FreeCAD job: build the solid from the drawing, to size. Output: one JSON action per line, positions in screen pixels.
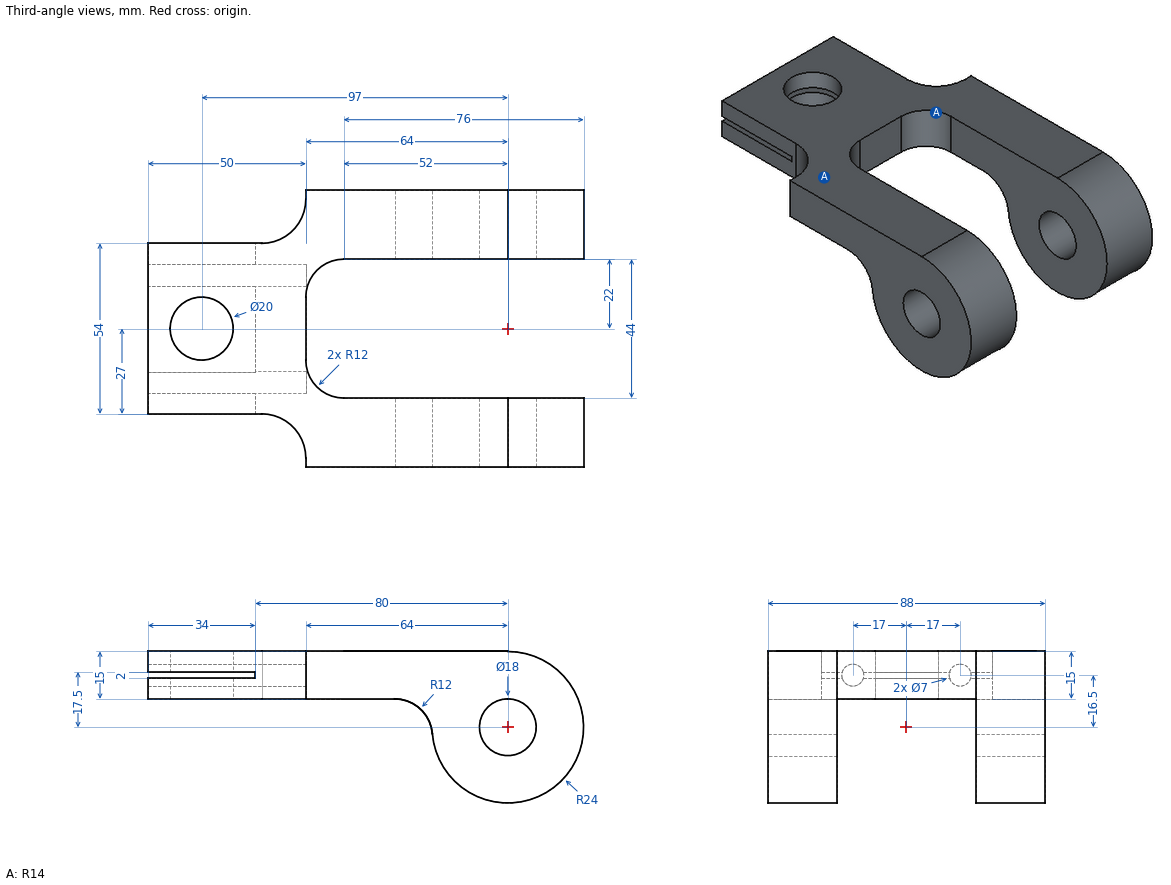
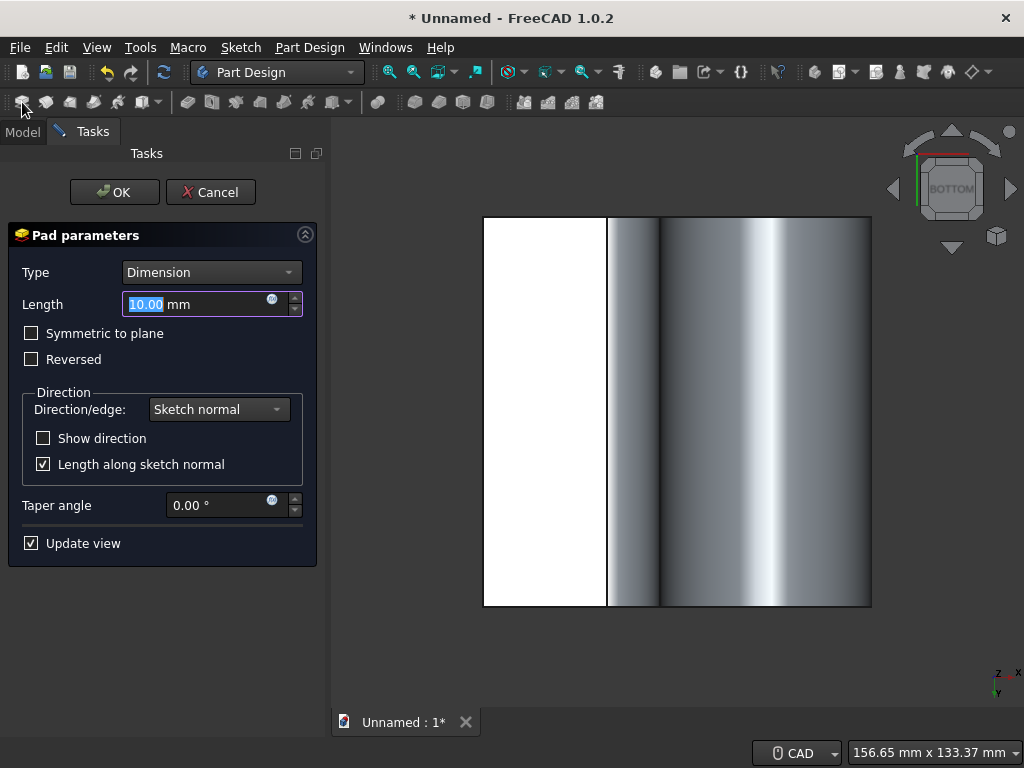
{"action": "type", "text": "15"}
{"action": "key", "text": "Tab"}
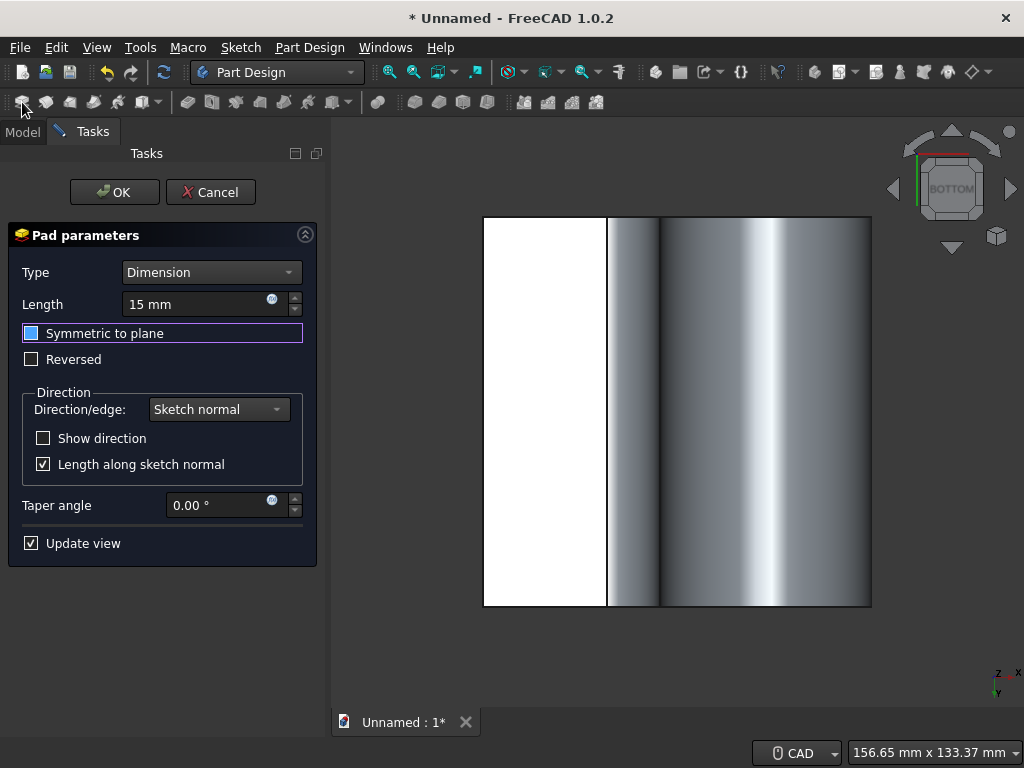
{"action": "left_click", "coordinate": [30, 359]}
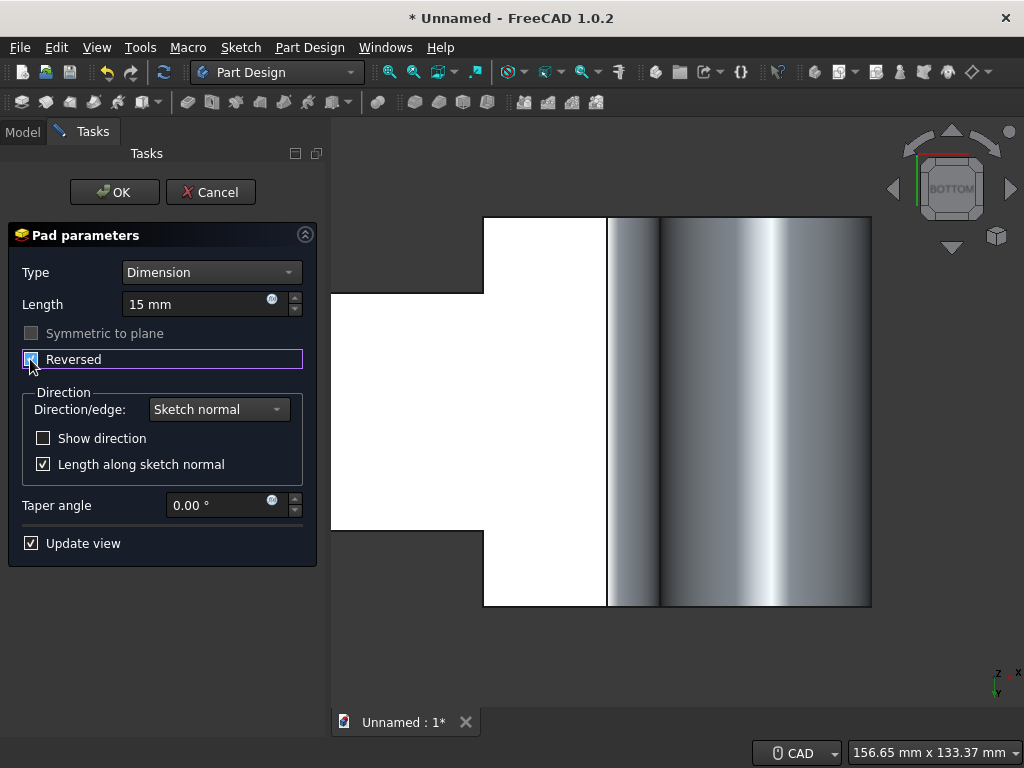
{"action": "left_click", "coordinate": [115, 192]}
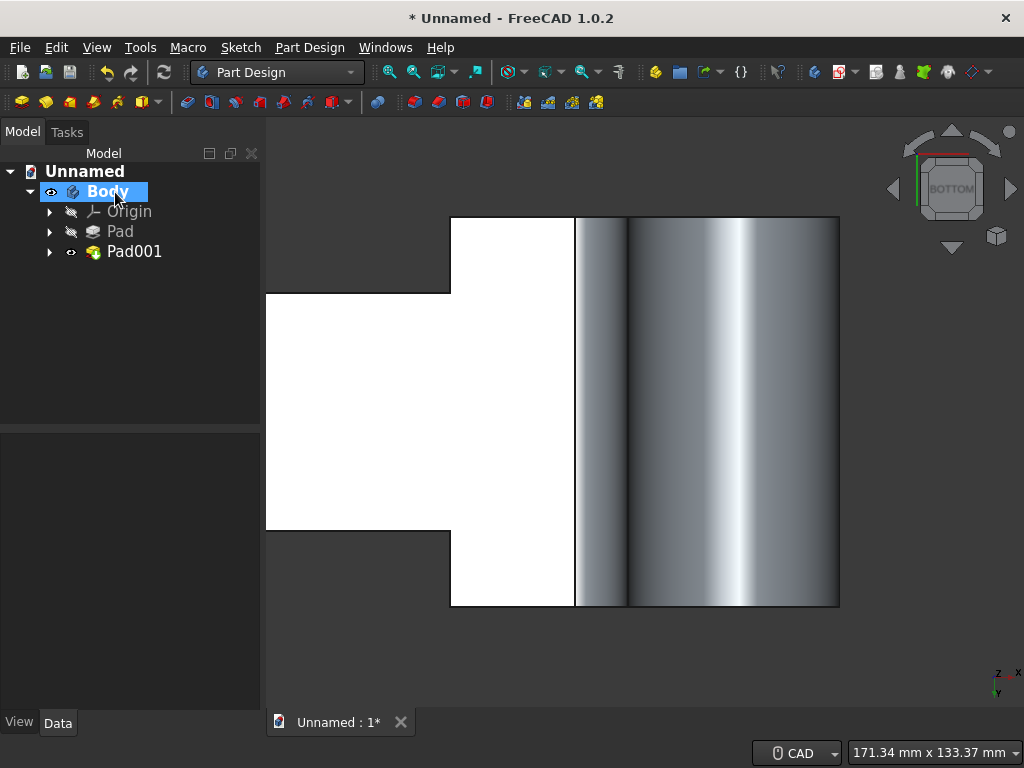
{"action": "left_click", "coordinate": [390, 72]}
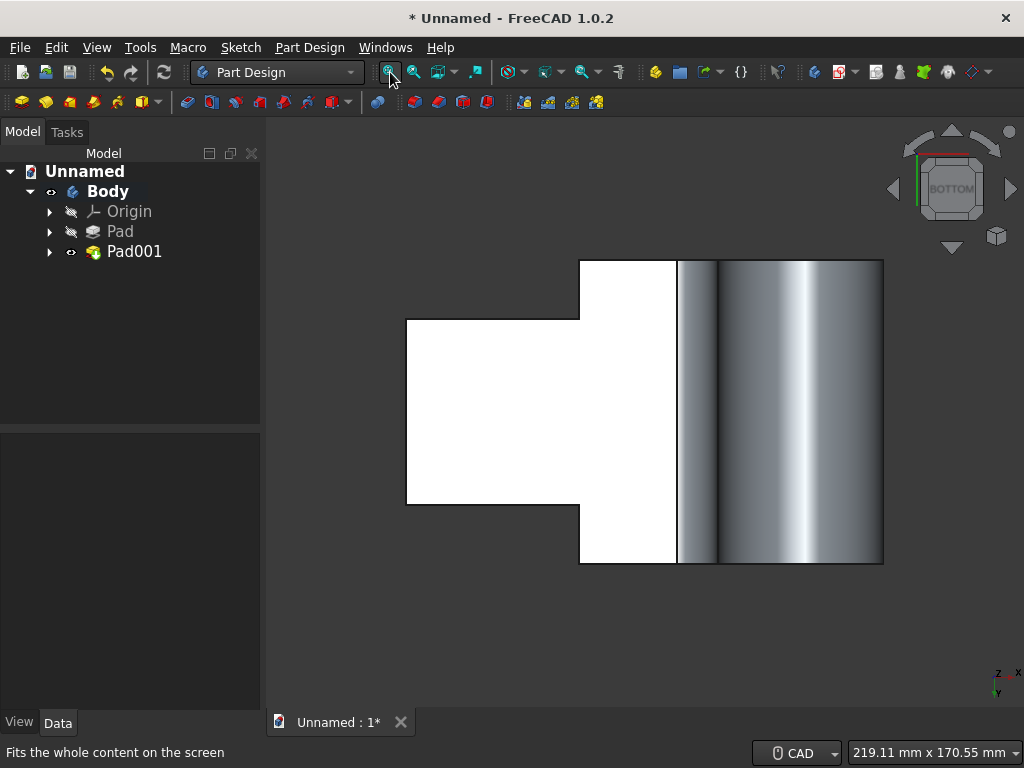
{"action": "left_click", "coordinate": [580, 411]}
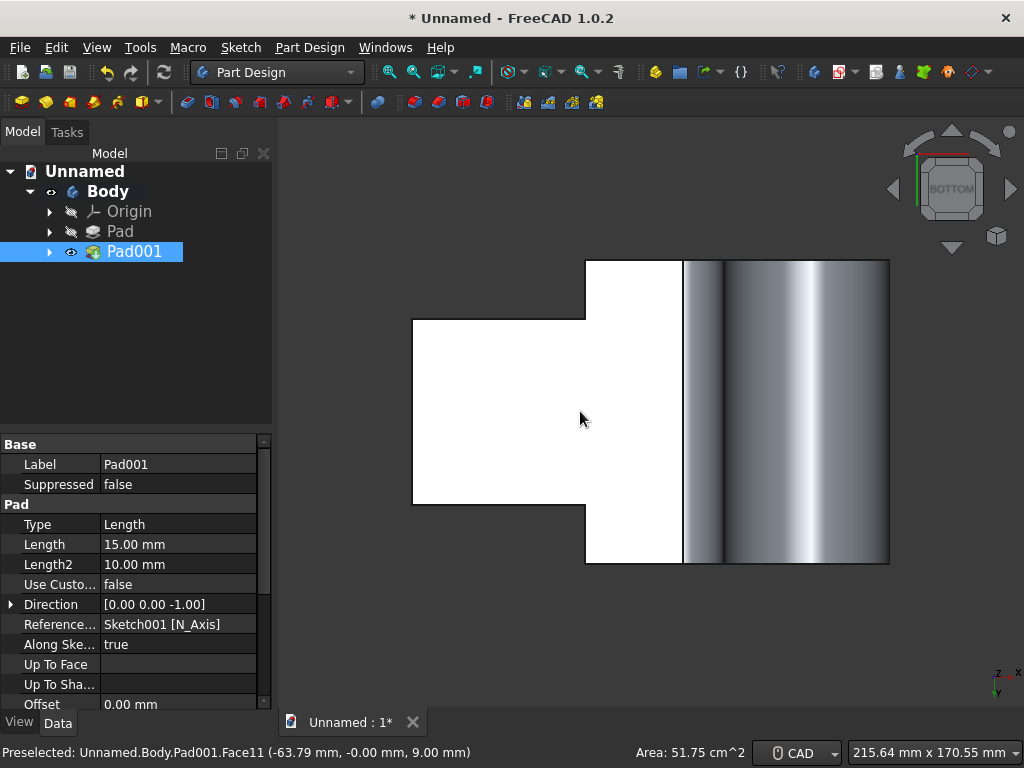
{"action": "left_click", "coordinate": [840, 72]}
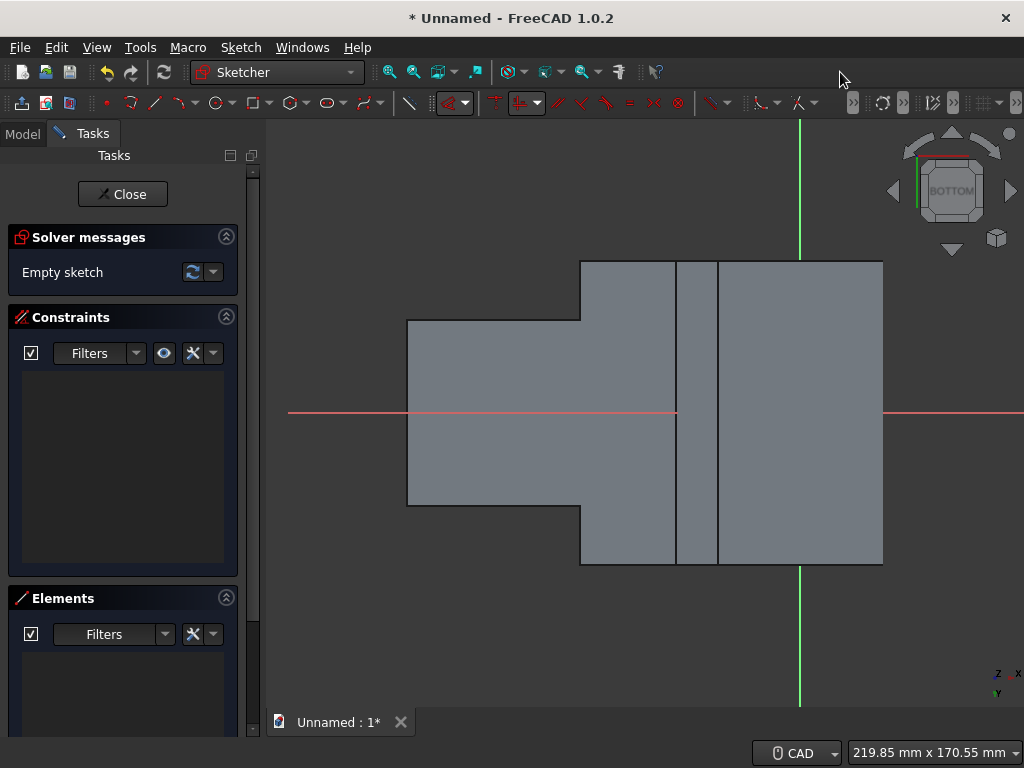
{"action": "left_click", "coordinate": [70, 104]}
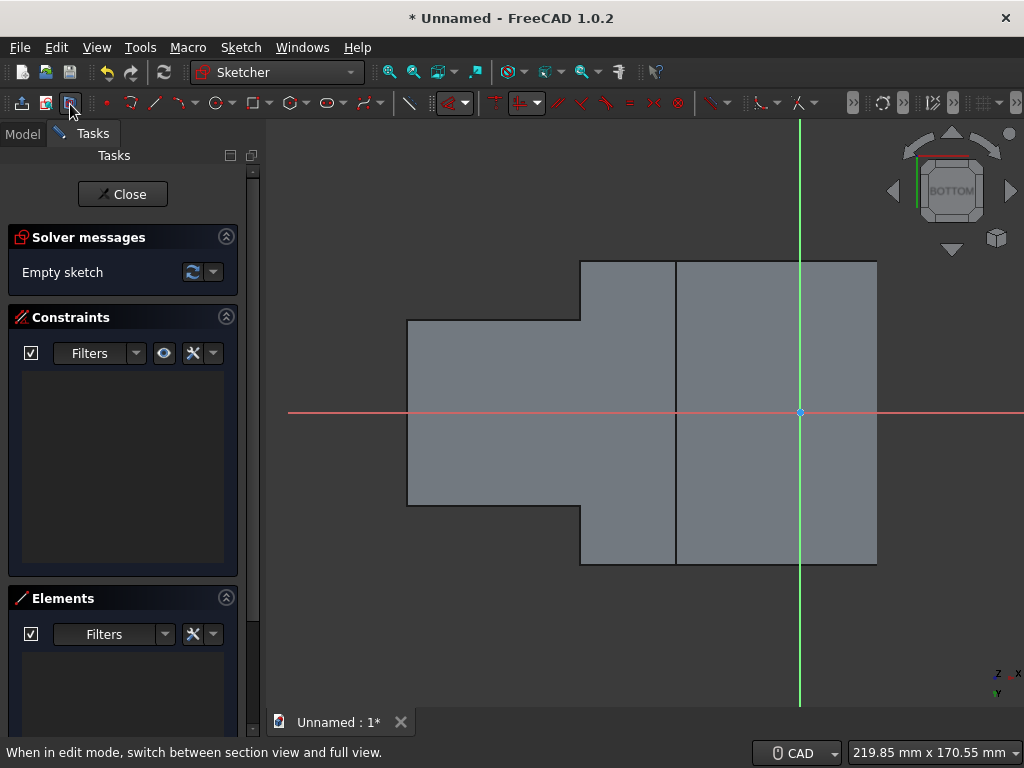
{"action": "scroll", "coordinate": [438, 413], "scroll_direction": "up", "scroll_amount": 8}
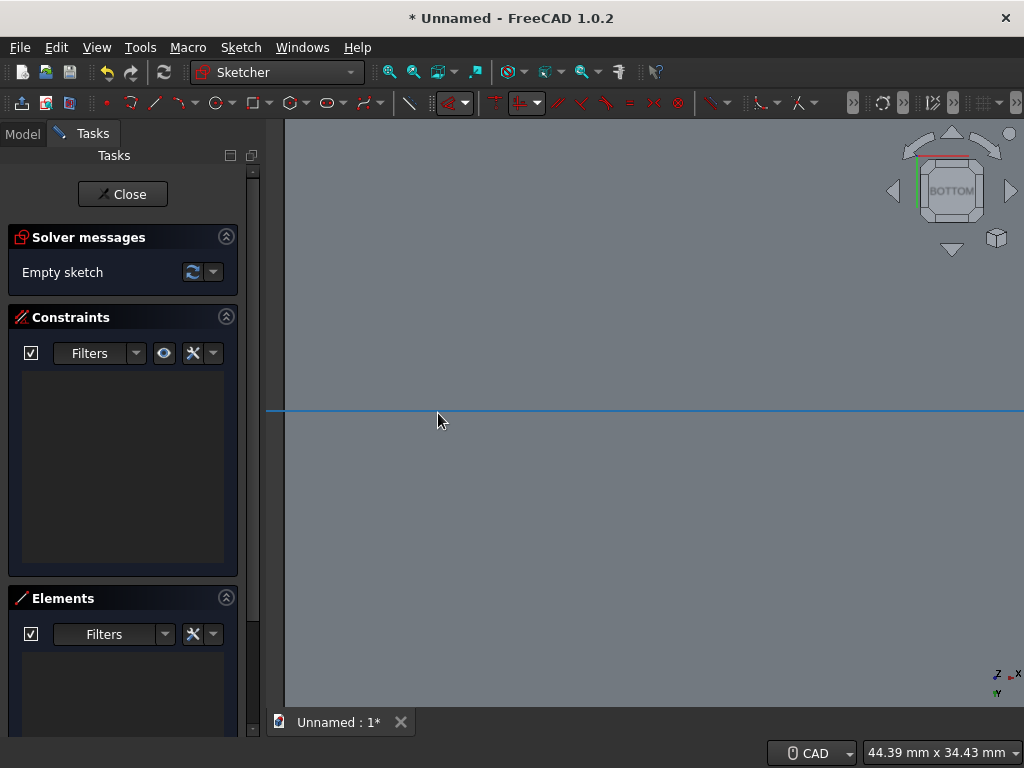
{"action": "left_click", "coordinate": [216, 104]}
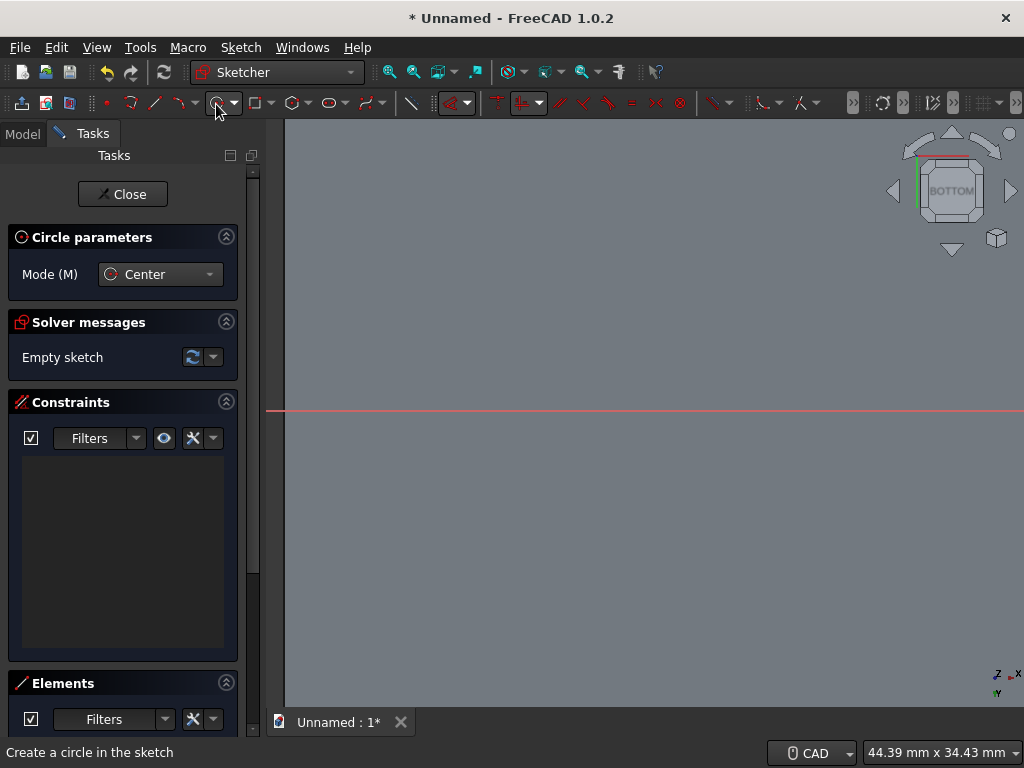
{"action": "left_click", "coordinate": [574, 411]}
{"action": "left_click", "coordinate": [695, 290]}
{"action": "key", "text": "Escape"}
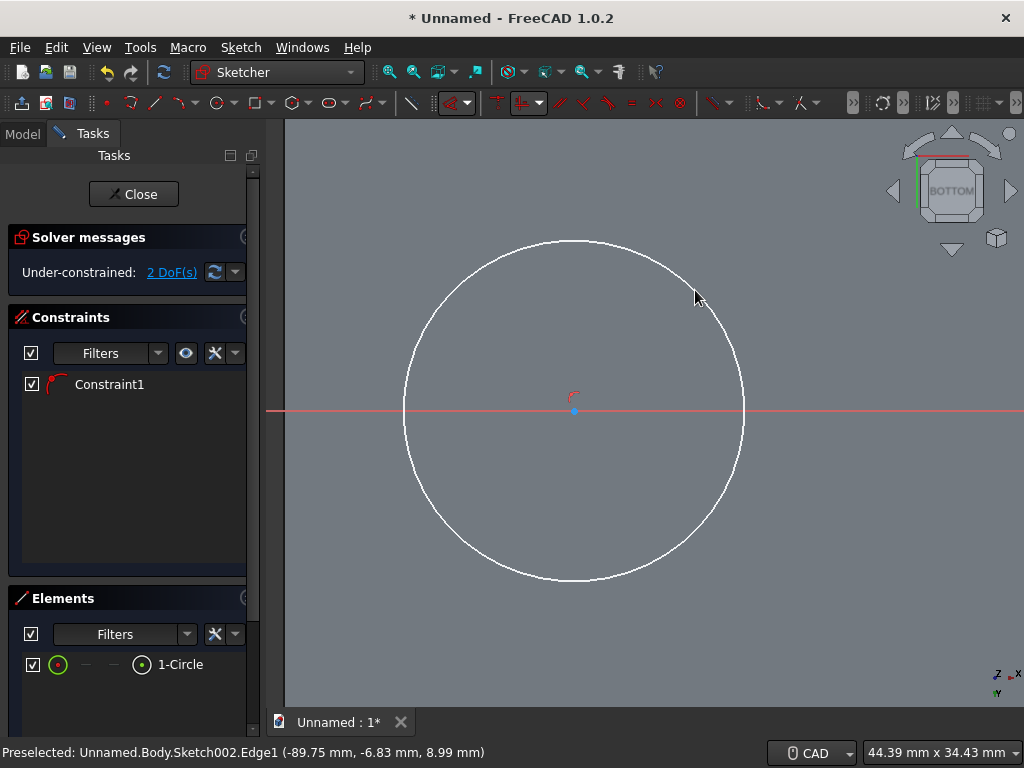
{"action": "left_click", "coordinate": [694, 290]}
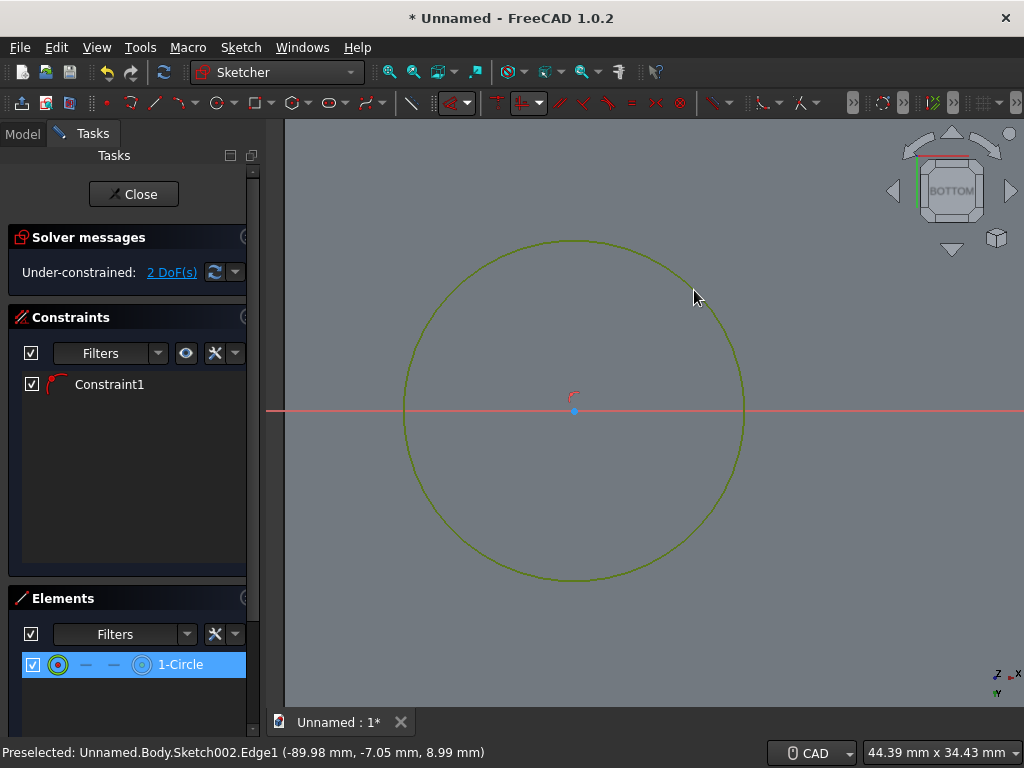
{"action": "left_click", "coordinate": [470, 104]}